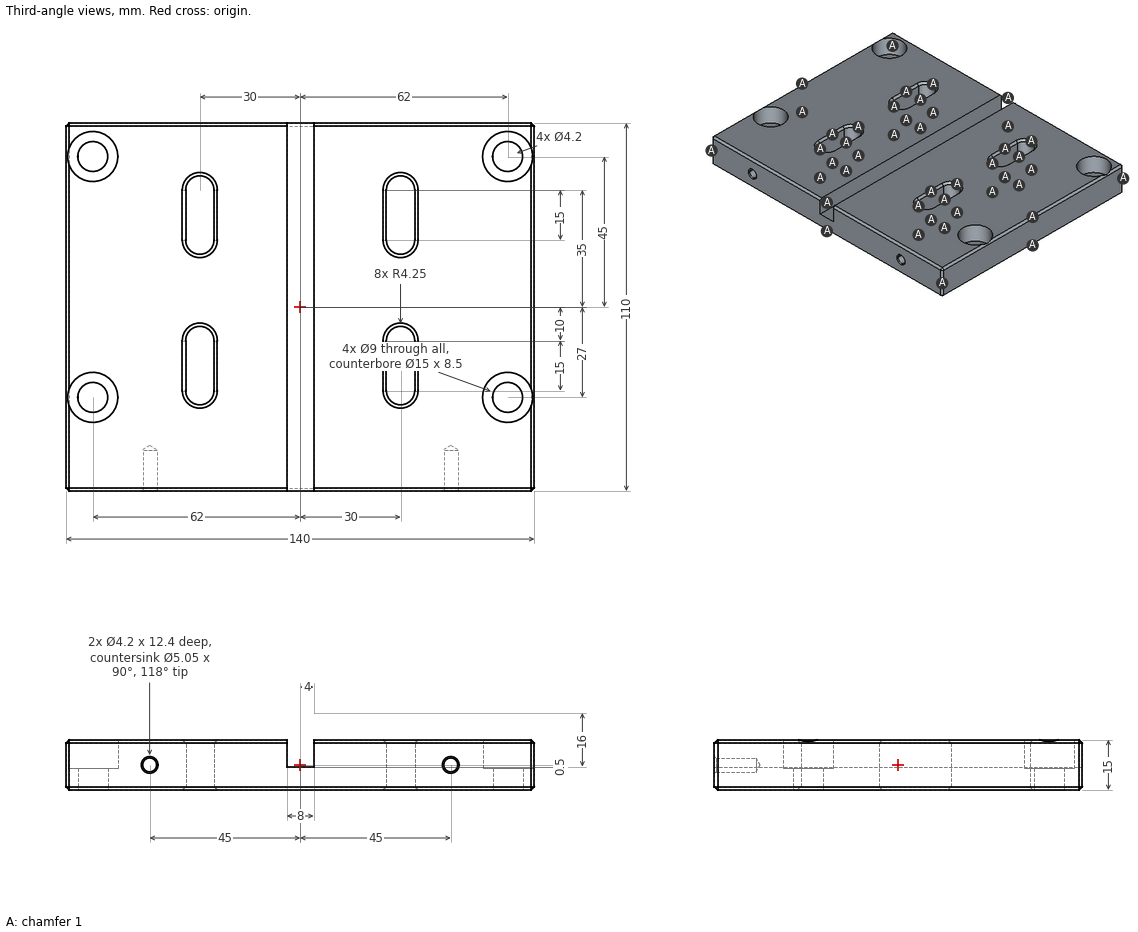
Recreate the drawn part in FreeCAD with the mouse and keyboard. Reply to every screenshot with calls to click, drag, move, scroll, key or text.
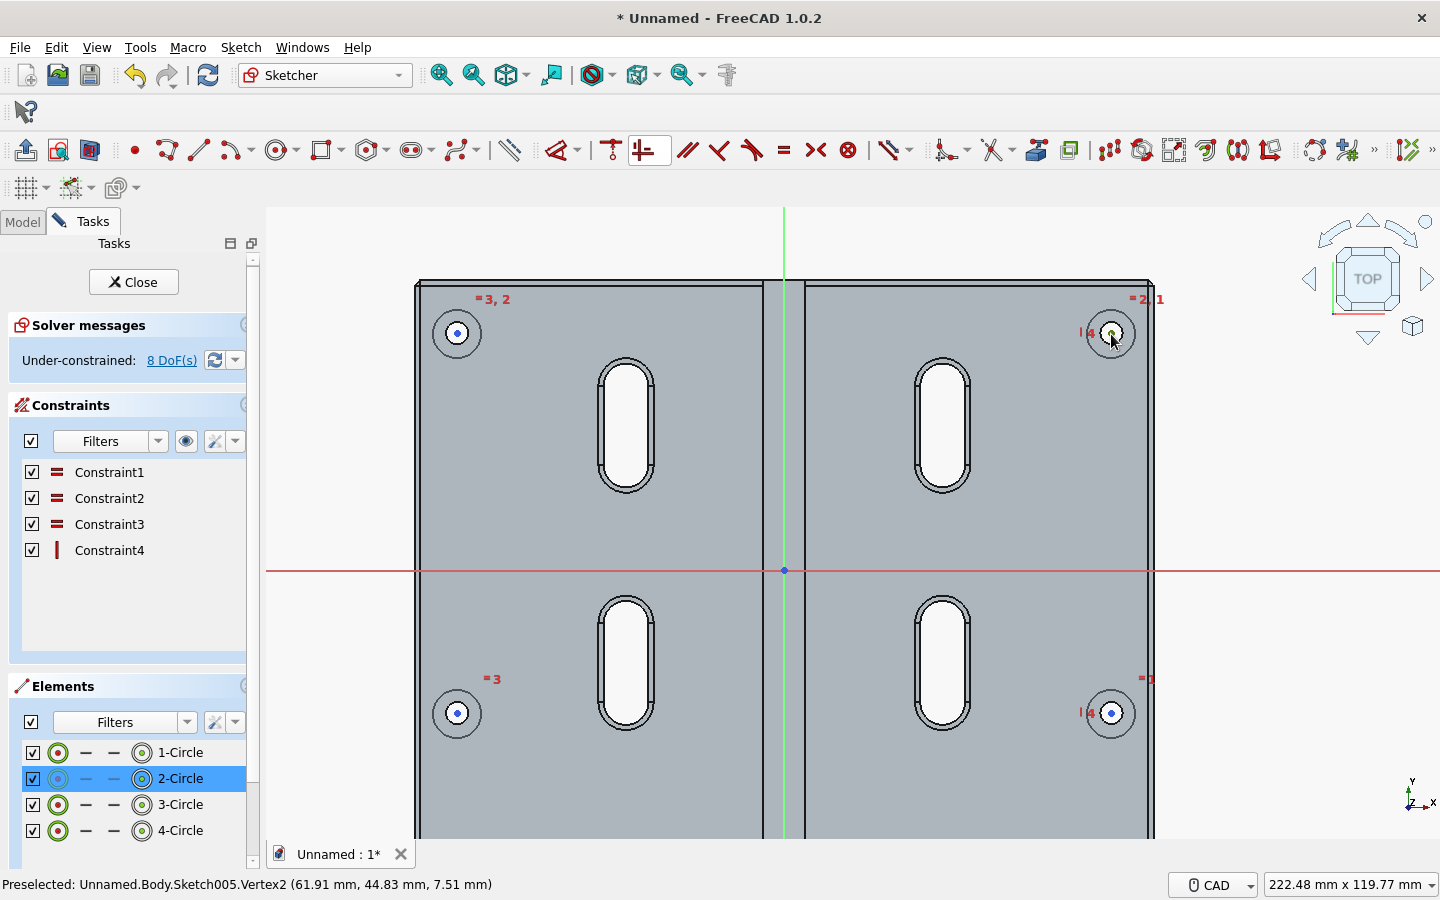
click(457, 334)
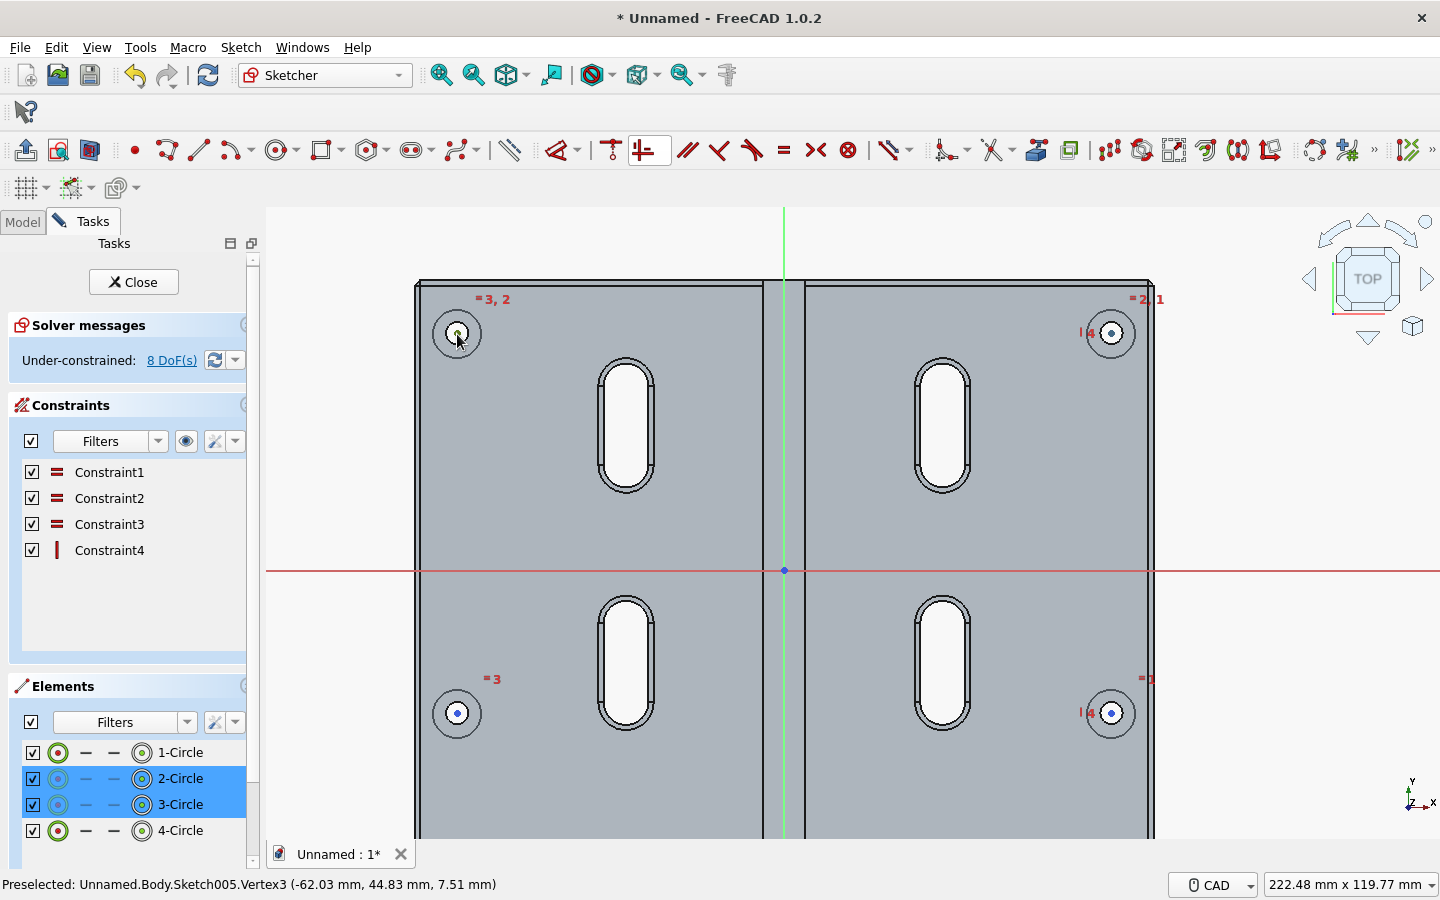
click(666, 150)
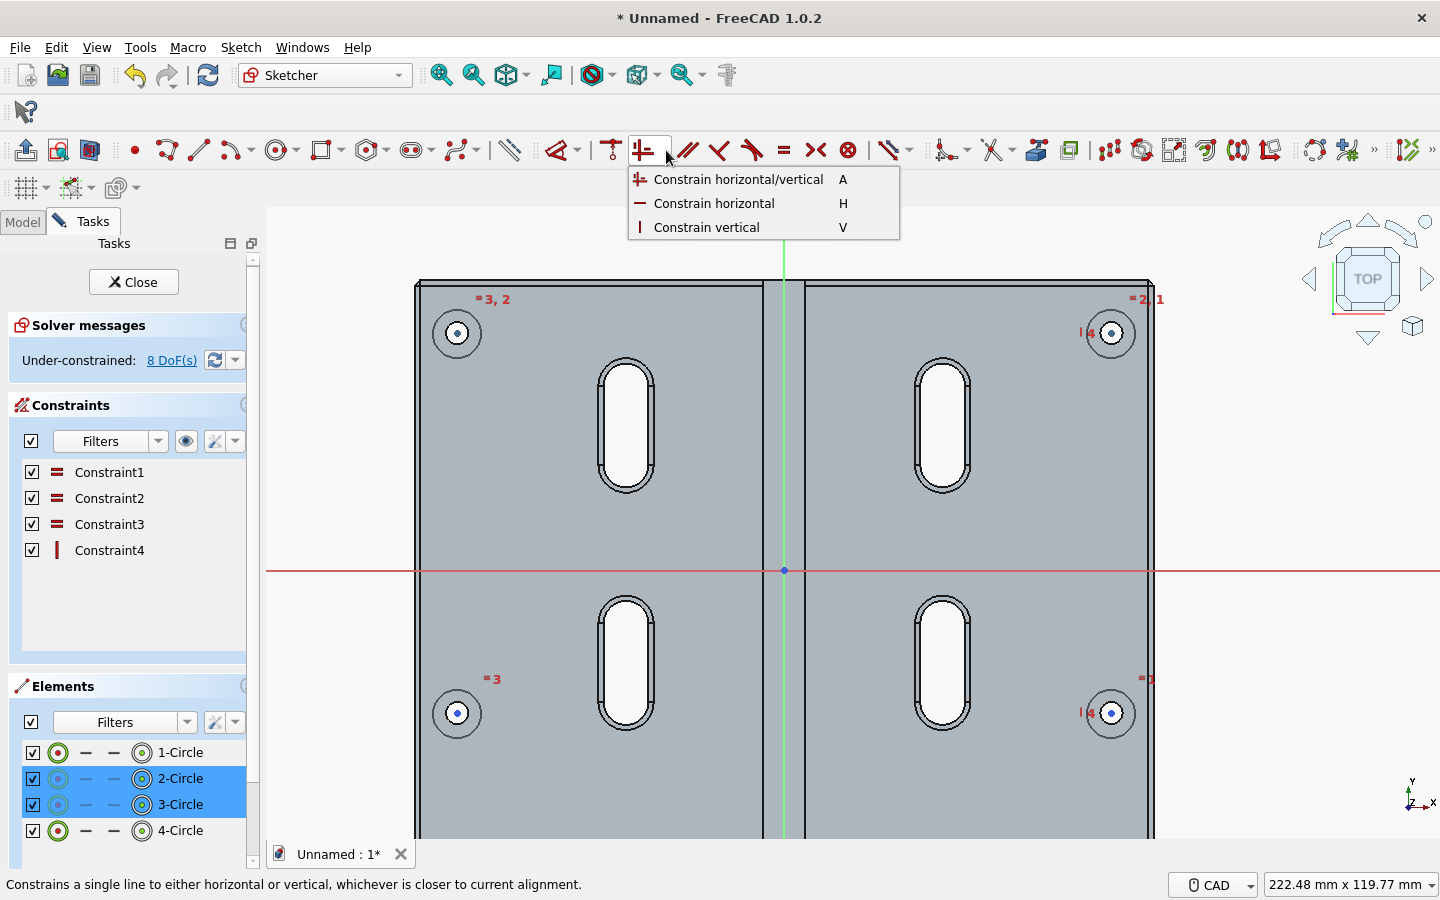
click(764, 203)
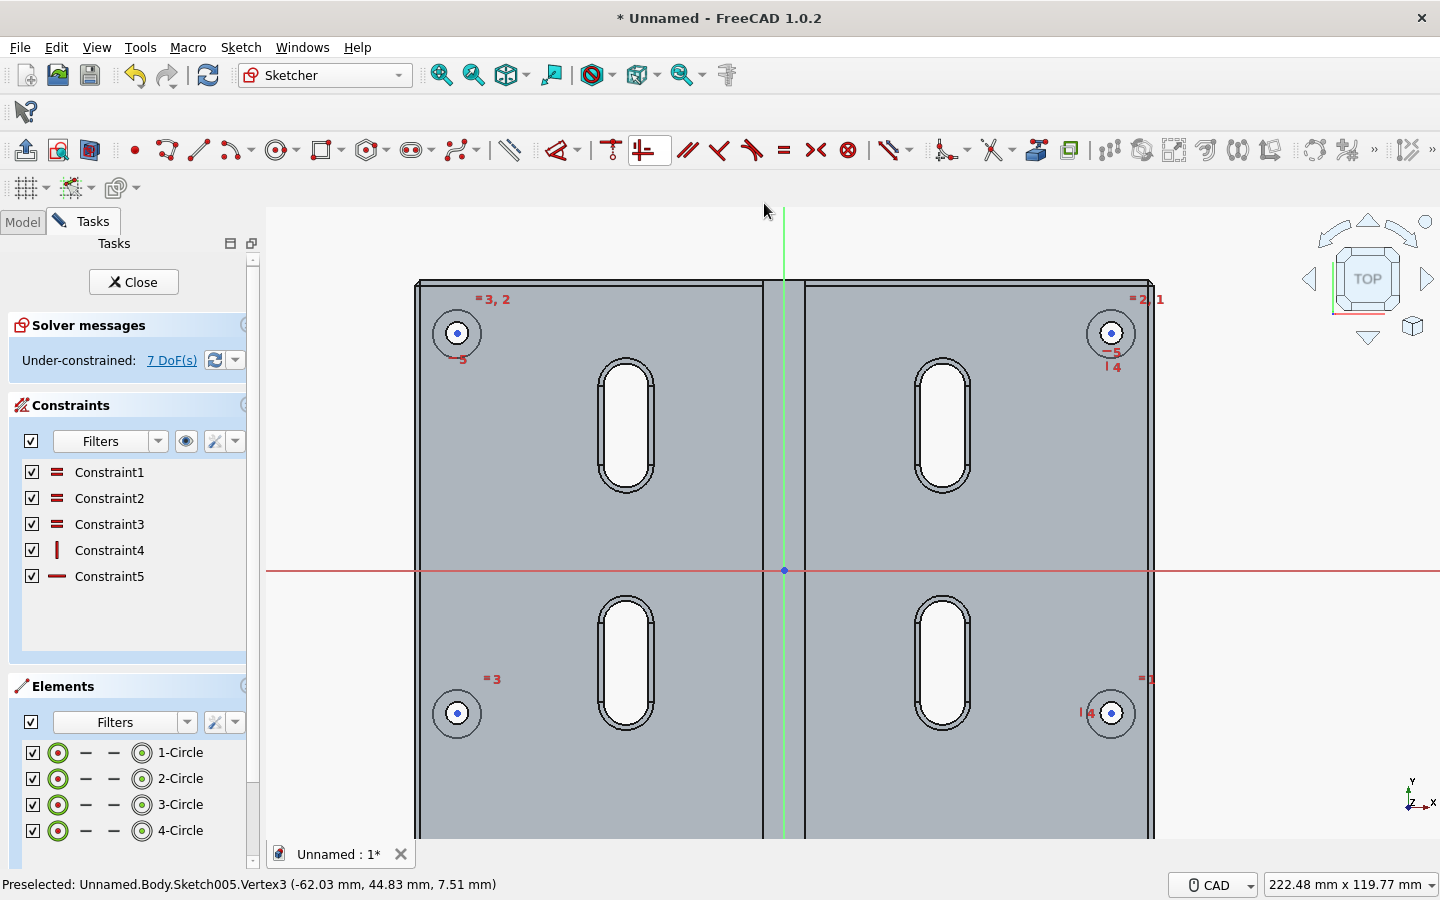
click(457, 334)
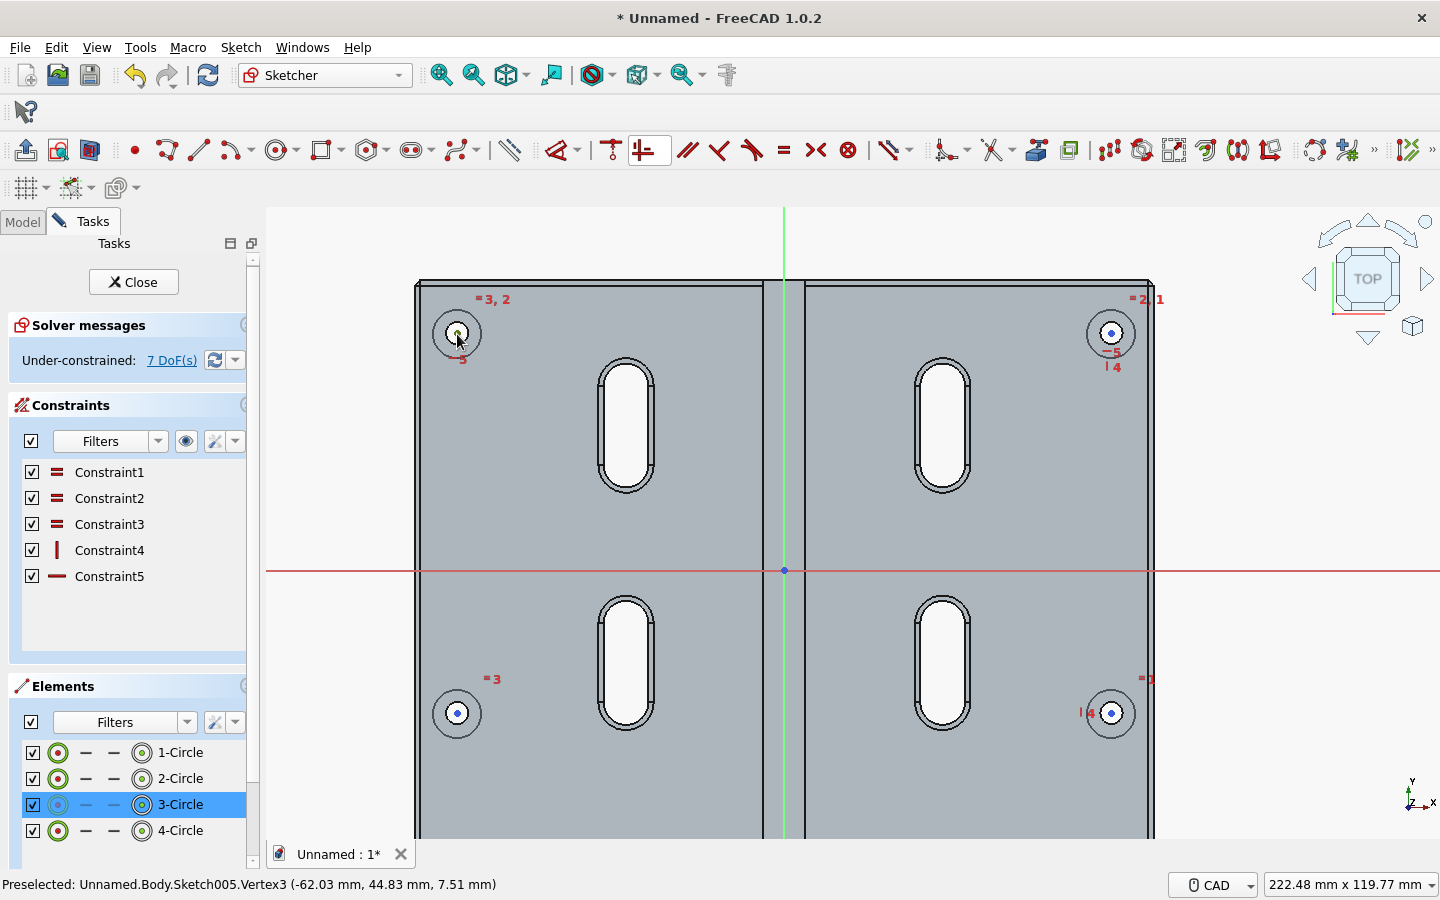
click(457, 714)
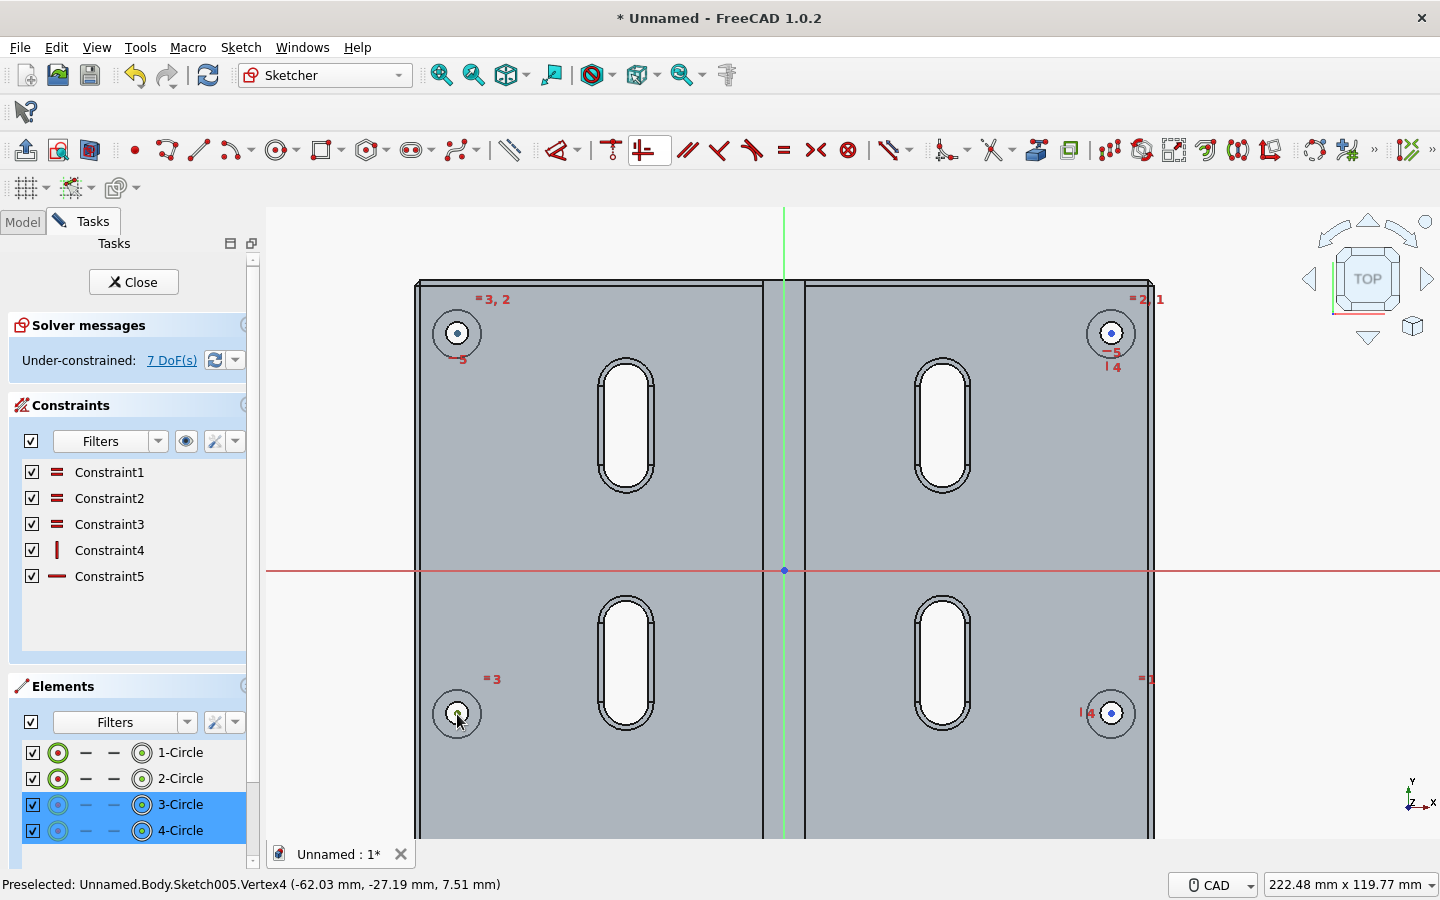
key(v)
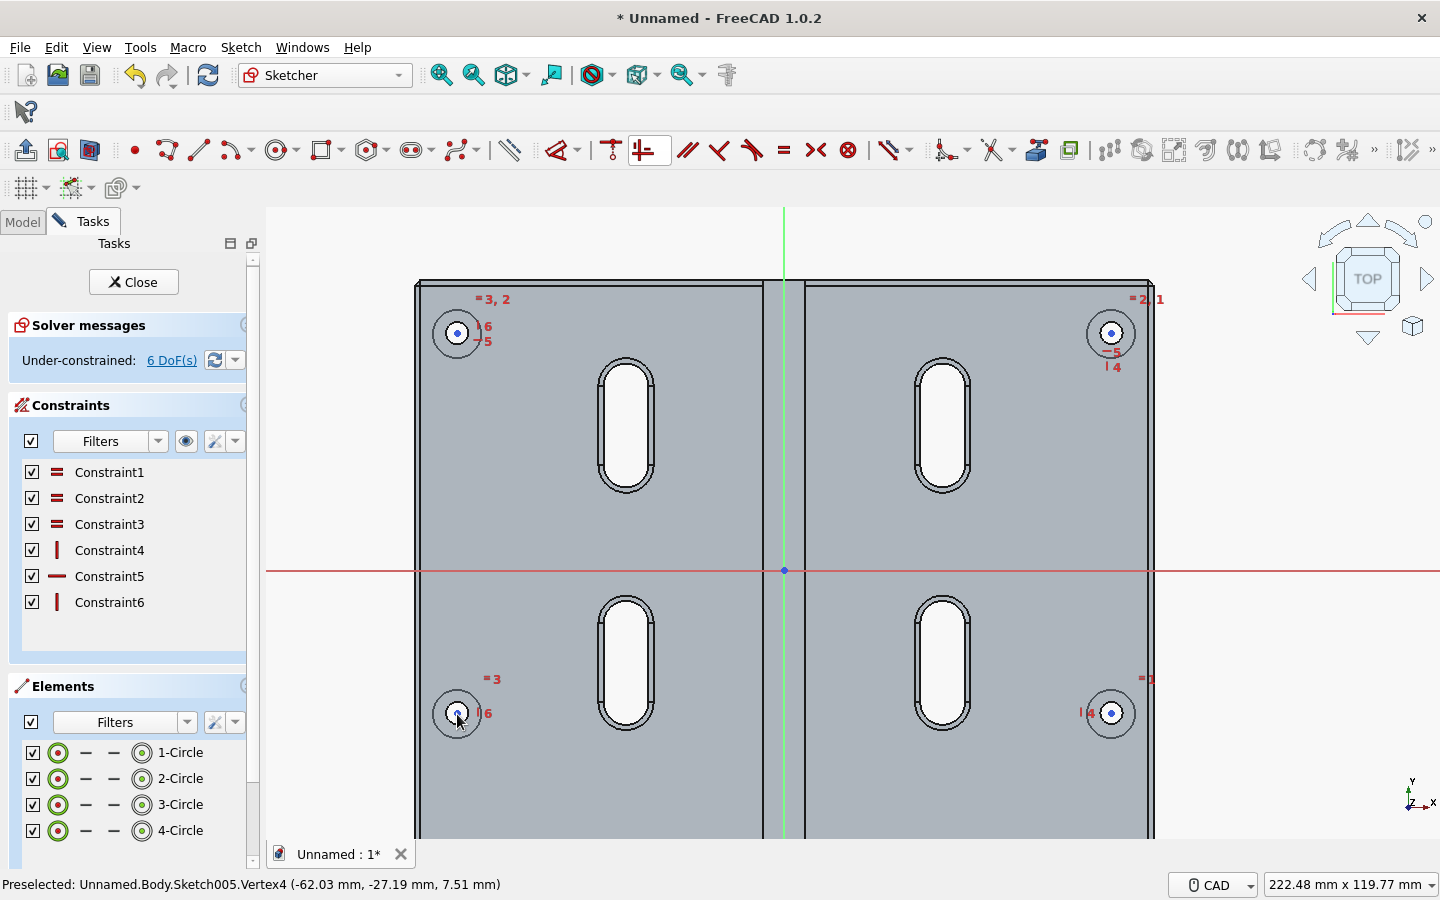
click(1111, 714)